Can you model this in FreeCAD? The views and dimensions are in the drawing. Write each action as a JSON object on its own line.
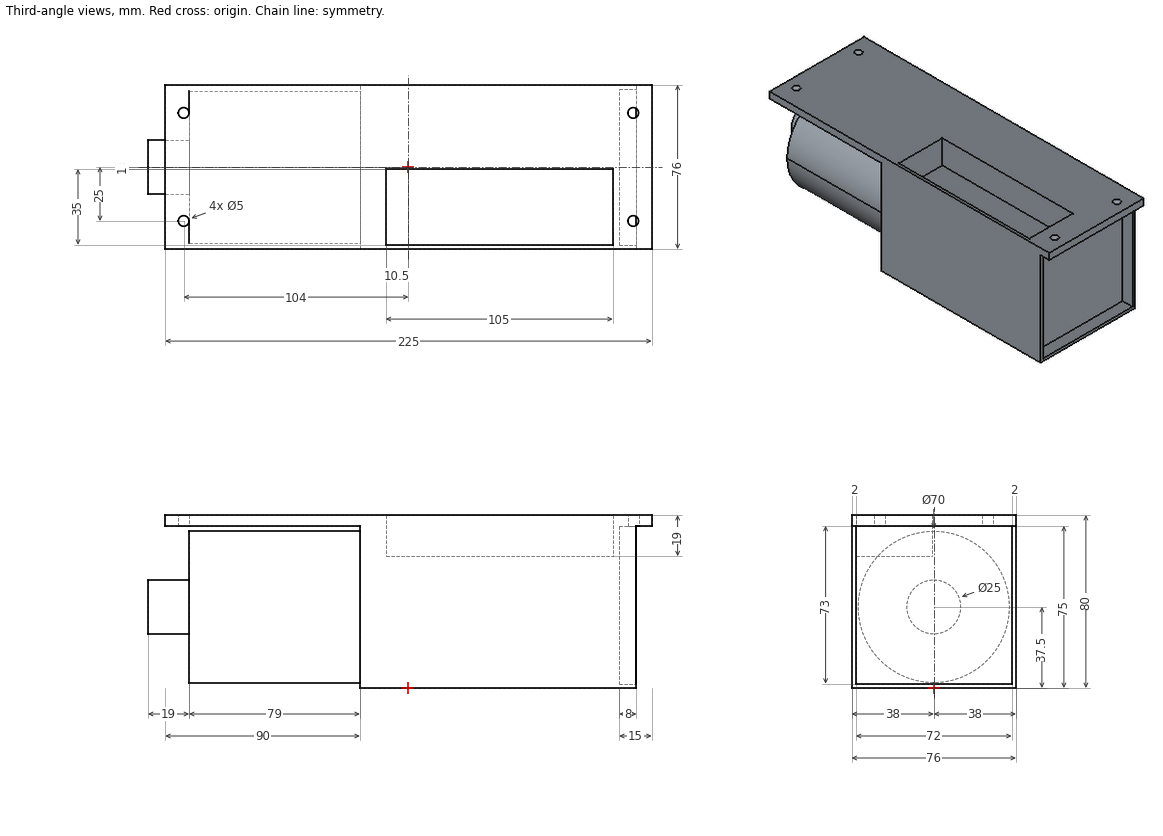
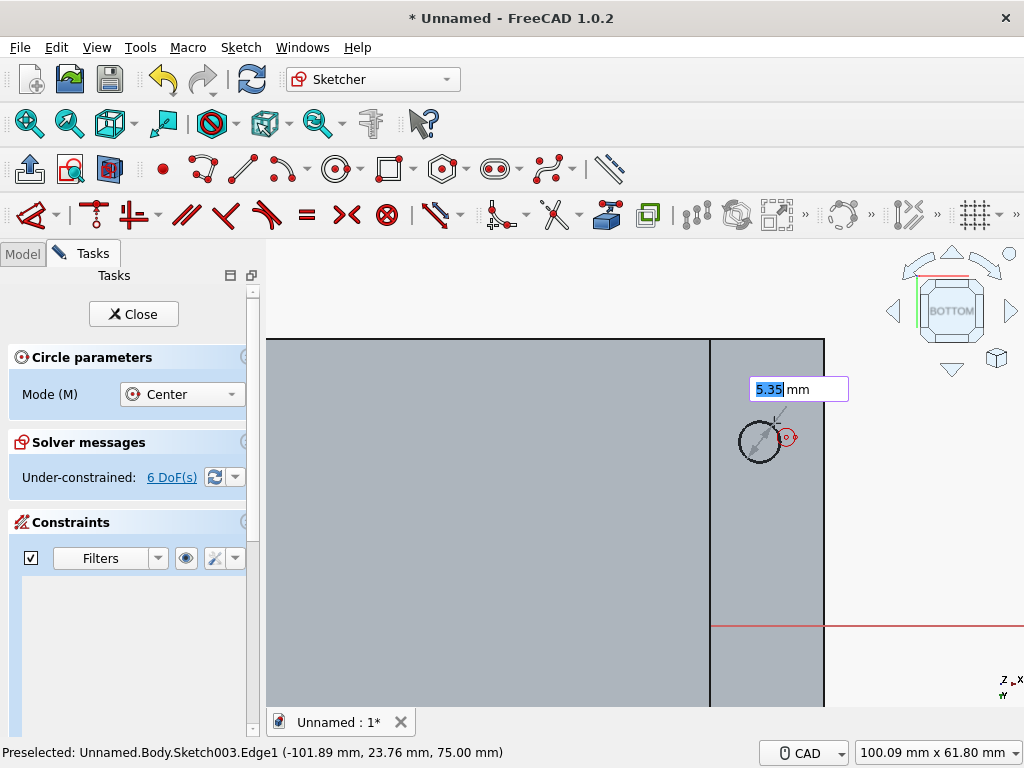
{"action": "left_click", "coordinate": [773, 424]}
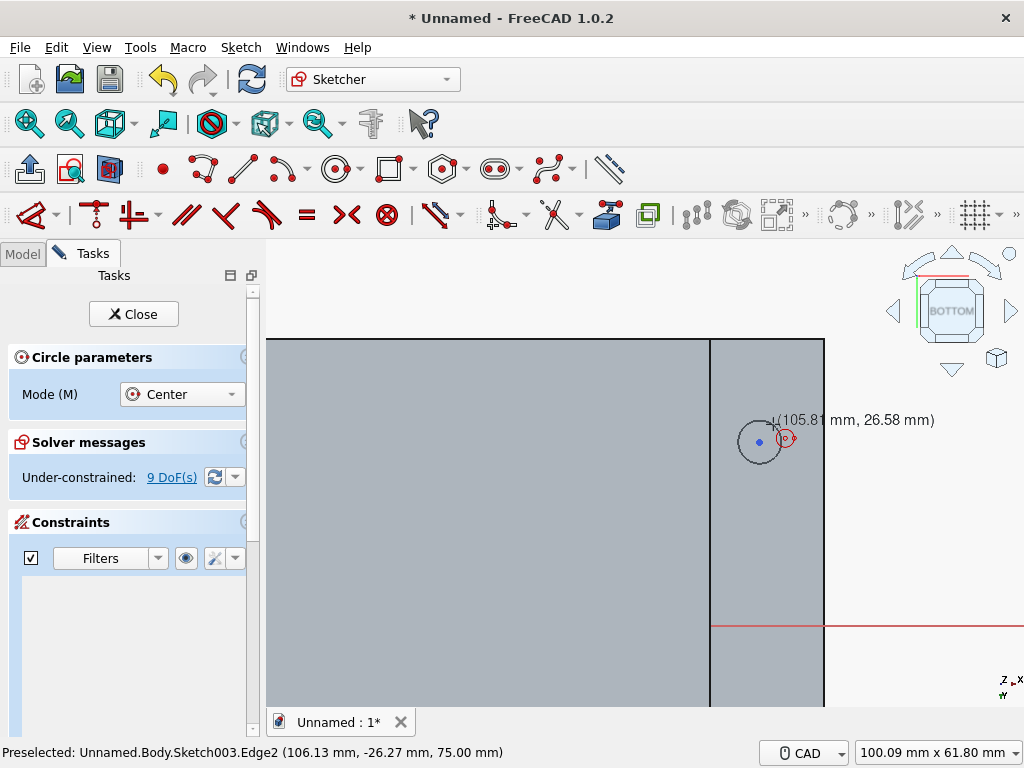
{"action": "scroll", "coordinate": [774, 423], "scroll_direction": "down", "scroll_amount": 7}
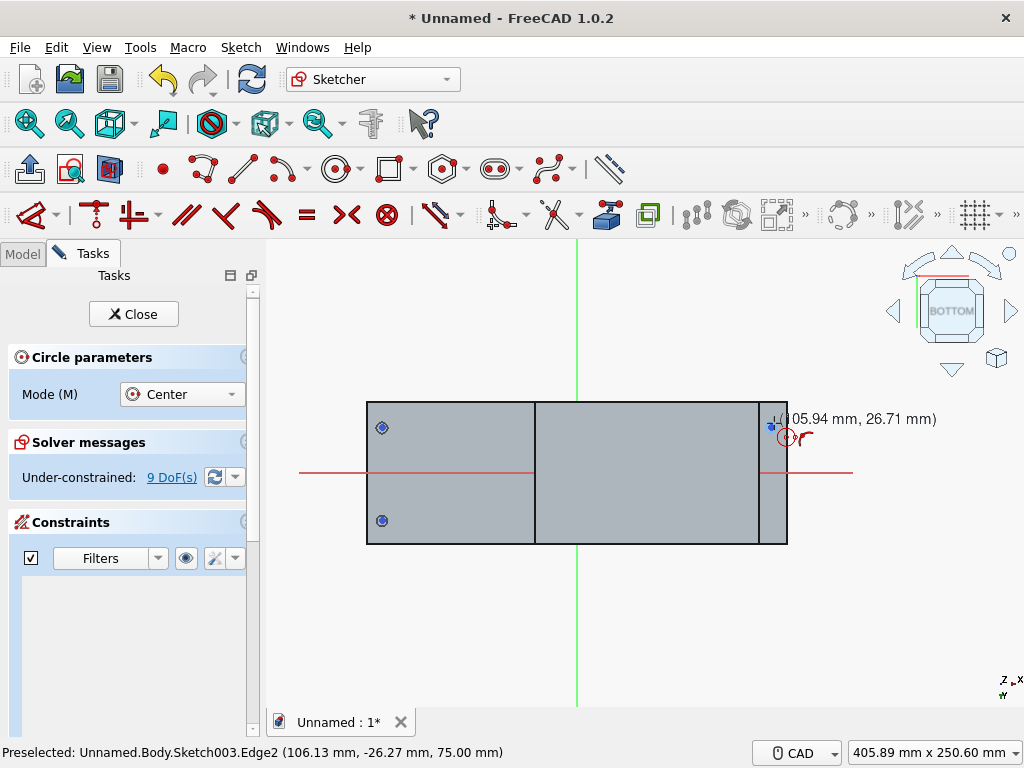
{"action": "scroll", "coordinate": [771, 520], "scroll_direction": "up", "scroll_amount": 8}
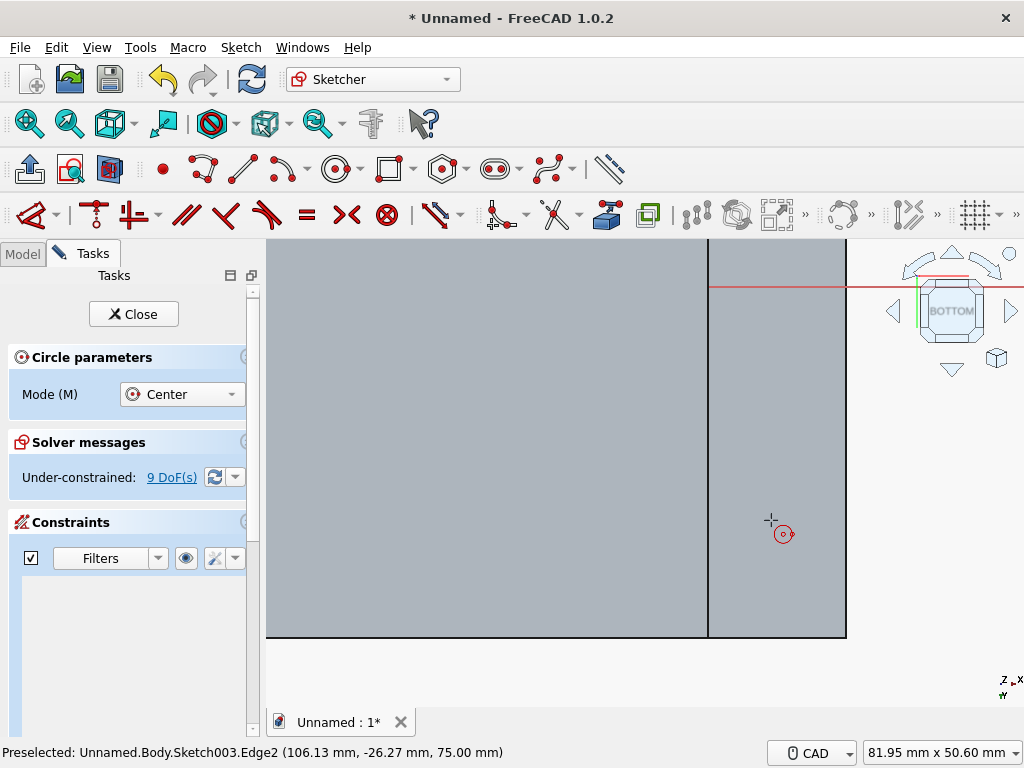
{"action": "scroll", "coordinate": [771, 520], "scroll_direction": "down", "scroll_amount": 8}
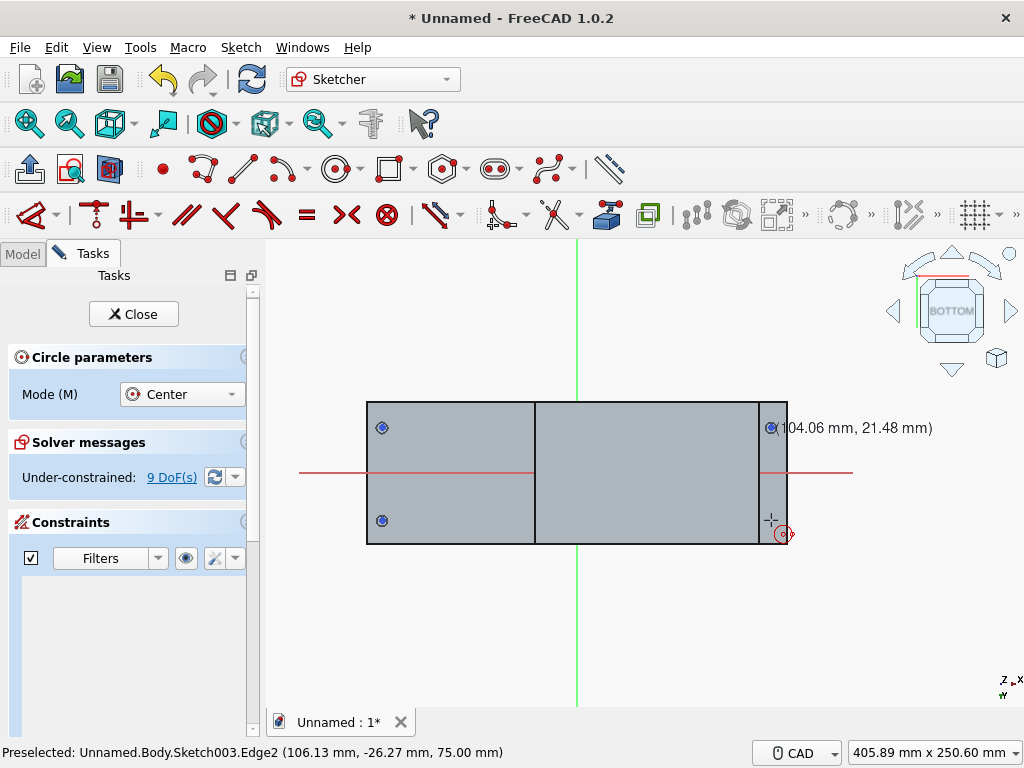
{"action": "left_click", "coordinate": [771, 520]}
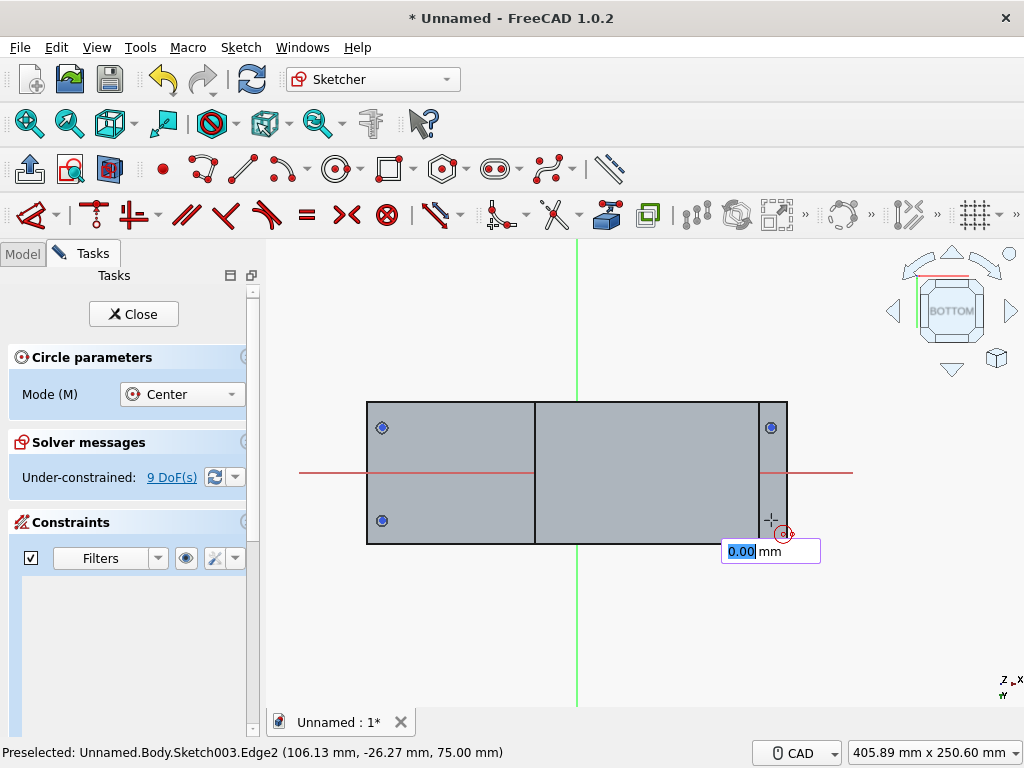
{"action": "scroll", "coordinate": [774, 517], "scroll_direction": "up", "scroll_amount": 7}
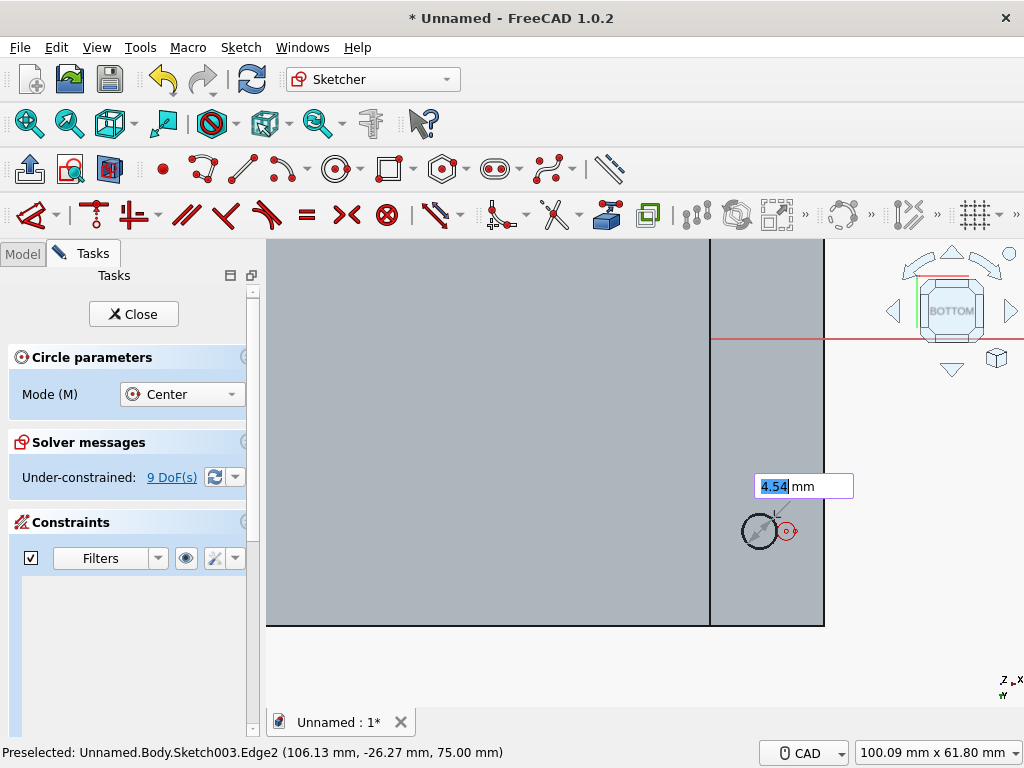
{"action": "left_click", "coordinate": [773, 514]}
{"action": "key", "text": "Escape"}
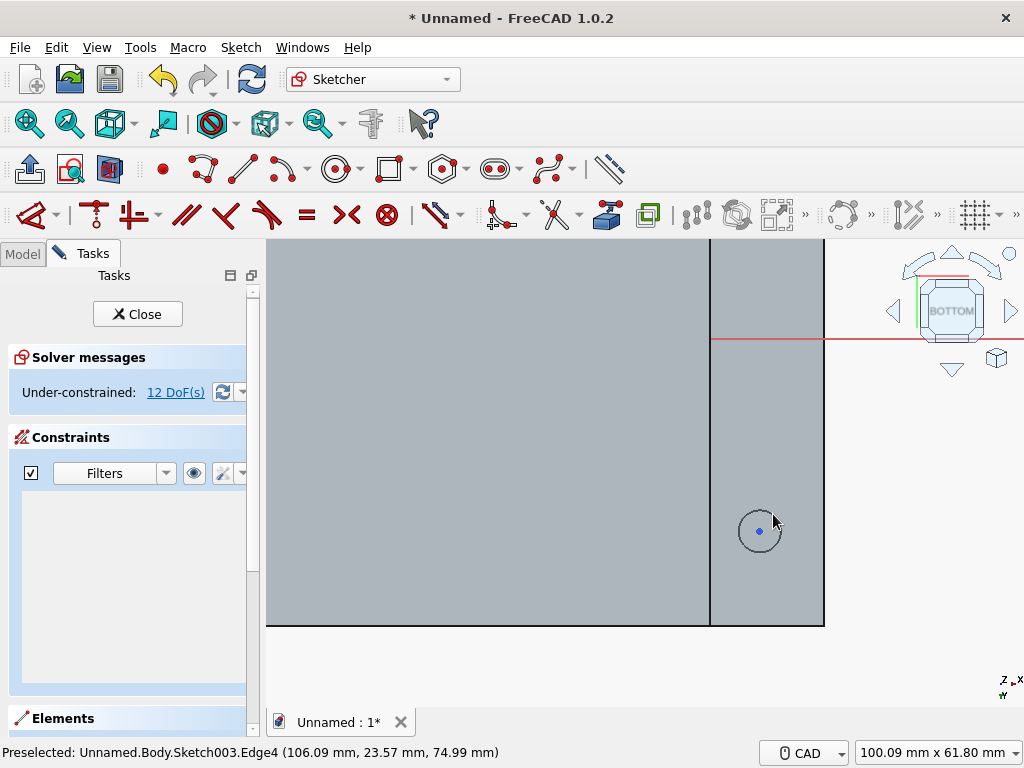
{"action": "scroll", "coordinate": [774, 517], "scroll_direction": "down", "scroll_amount": 7}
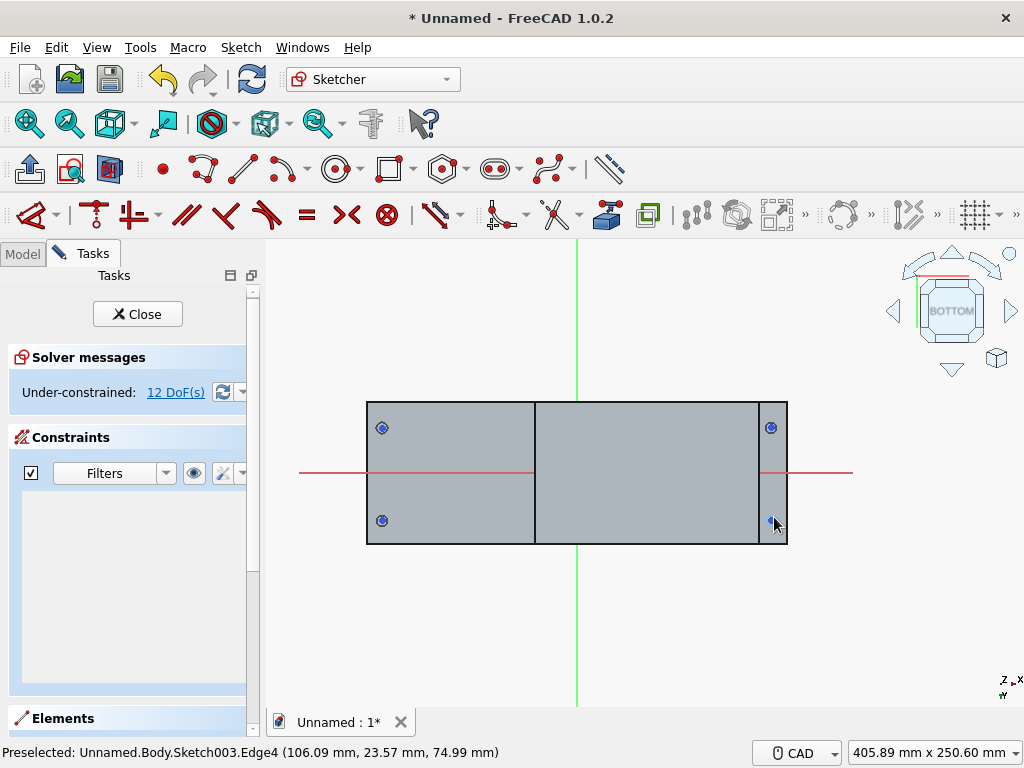
{"action": "scroll", "coordinate": [386, 424], "scroll_direction": "up", "scroll_amount": 5}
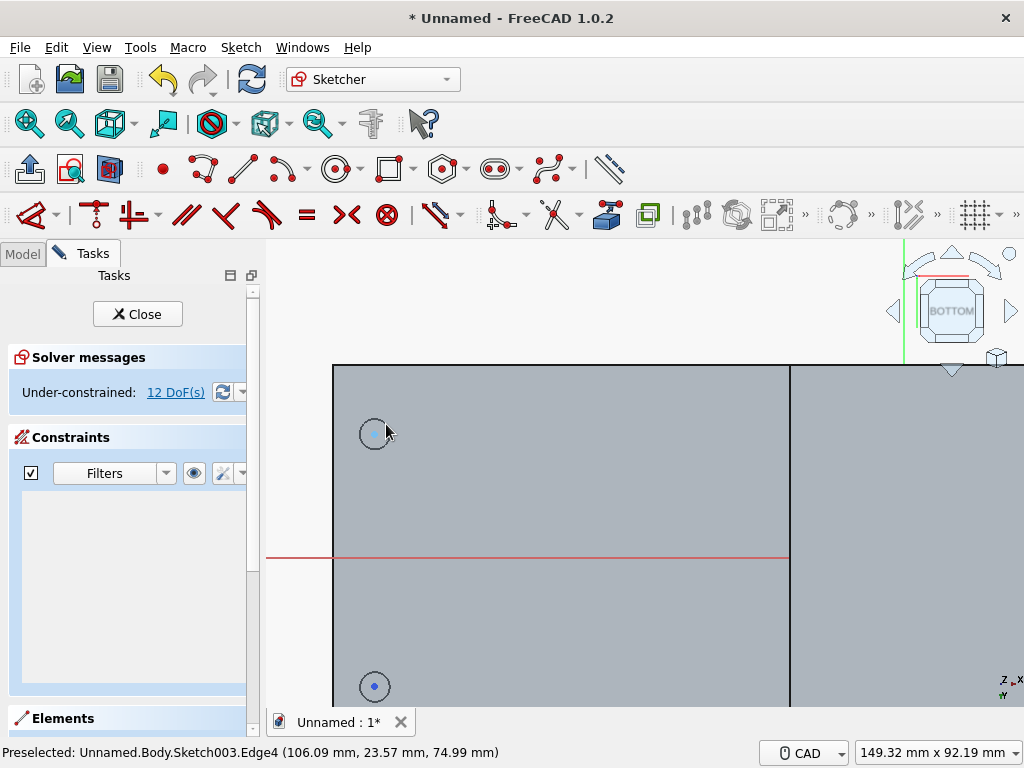
{"action": "left_click", "coordinate": [386, 423]}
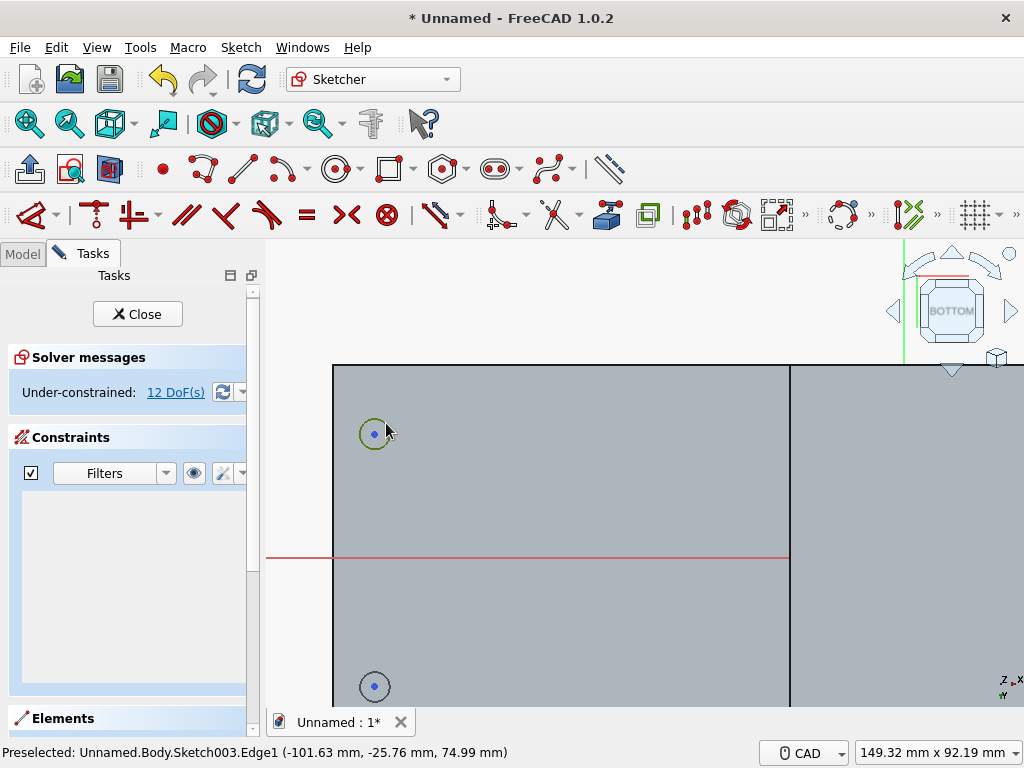
{"action": "left_click", "coordinate": [385, 677]}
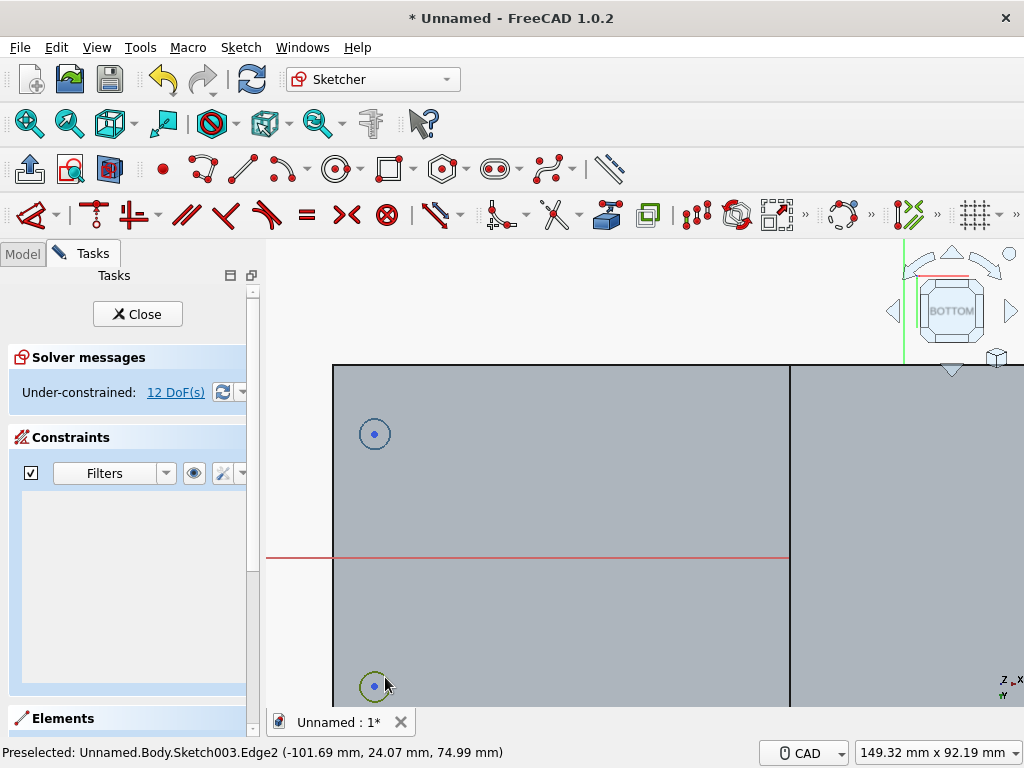
{"action": "scroll", "coordinate": [386, 424], "scroll_direction": "down", "scroll_amount": 5}